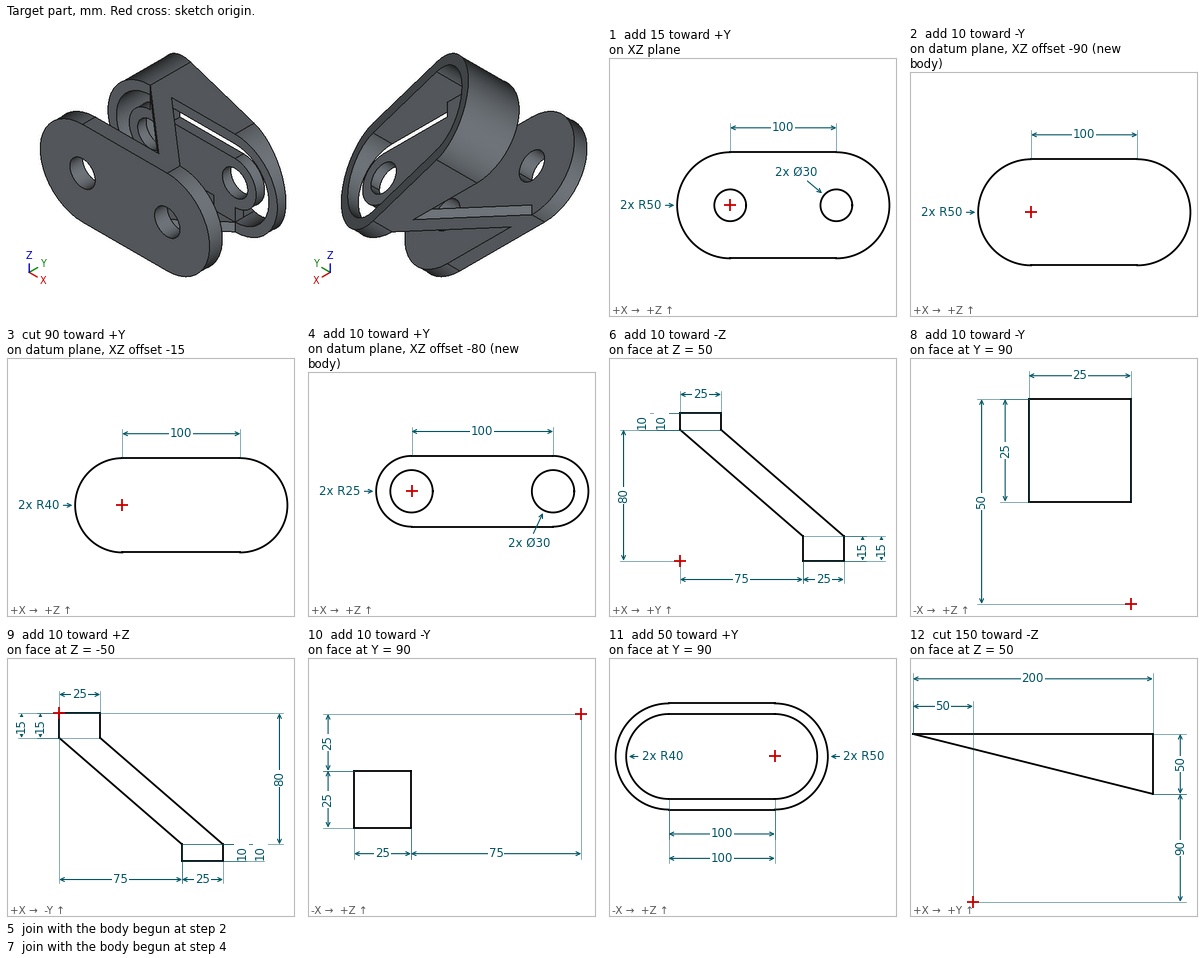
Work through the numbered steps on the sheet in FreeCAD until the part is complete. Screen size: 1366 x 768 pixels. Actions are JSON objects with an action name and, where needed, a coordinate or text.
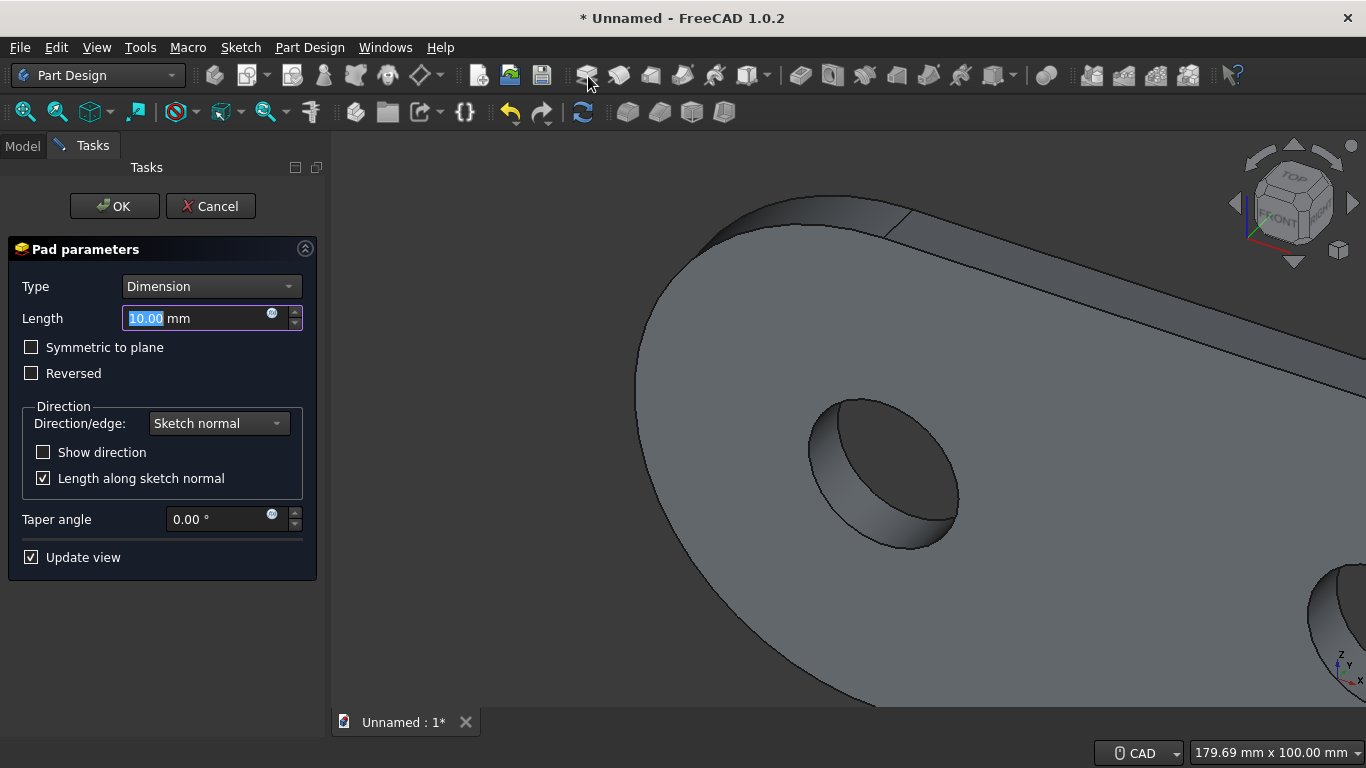
{"action": "type", "text": "15"}
{"action": "key", "text": "Tab"}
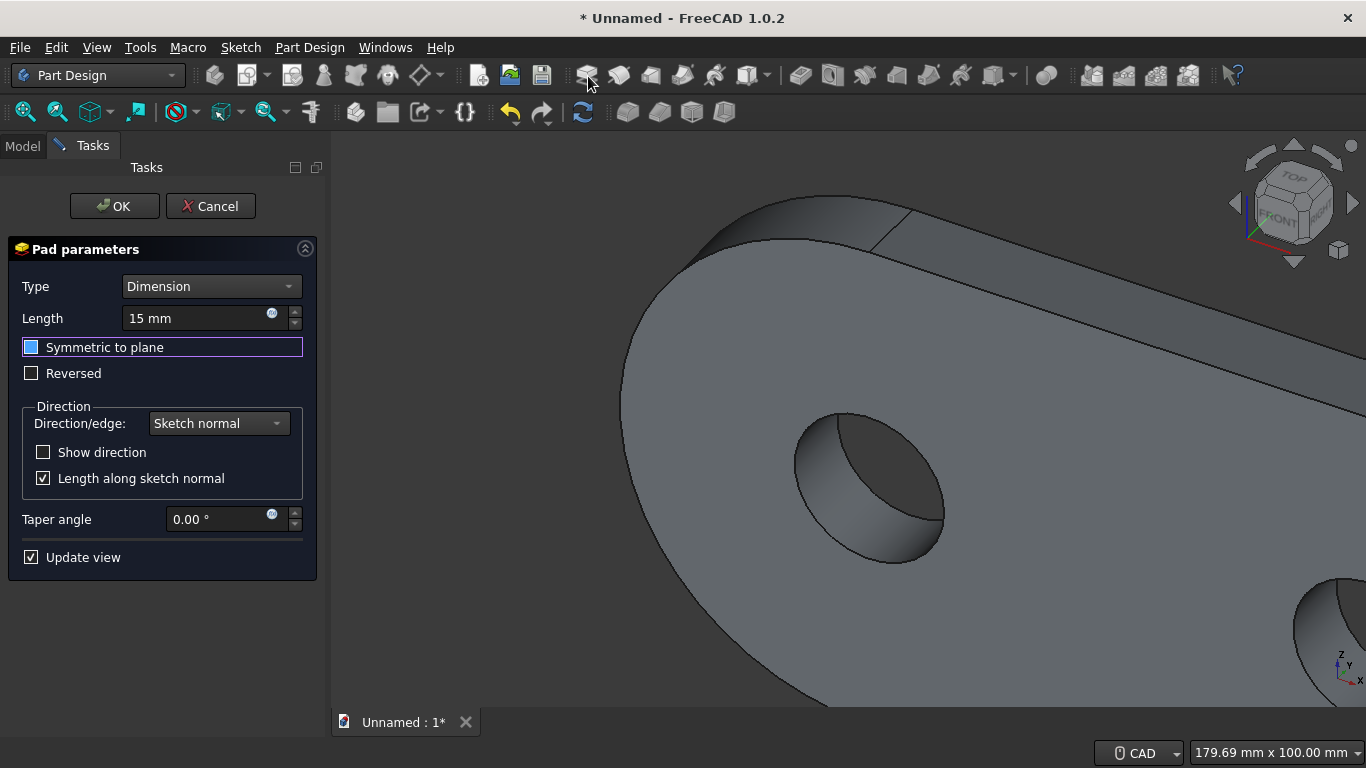
{"action": "left_click", "coordinate": [30, 373]}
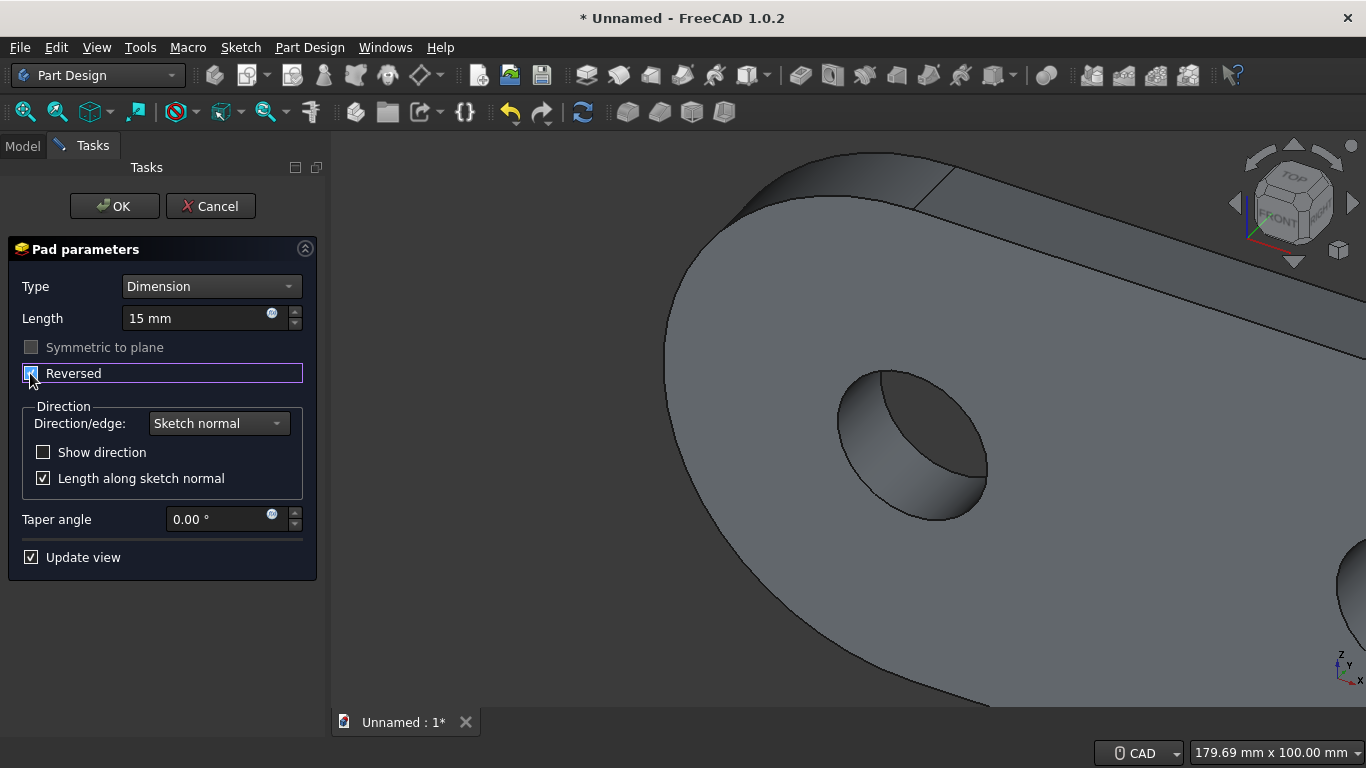
{"action": "left_click", "coordinate": [115, 206]}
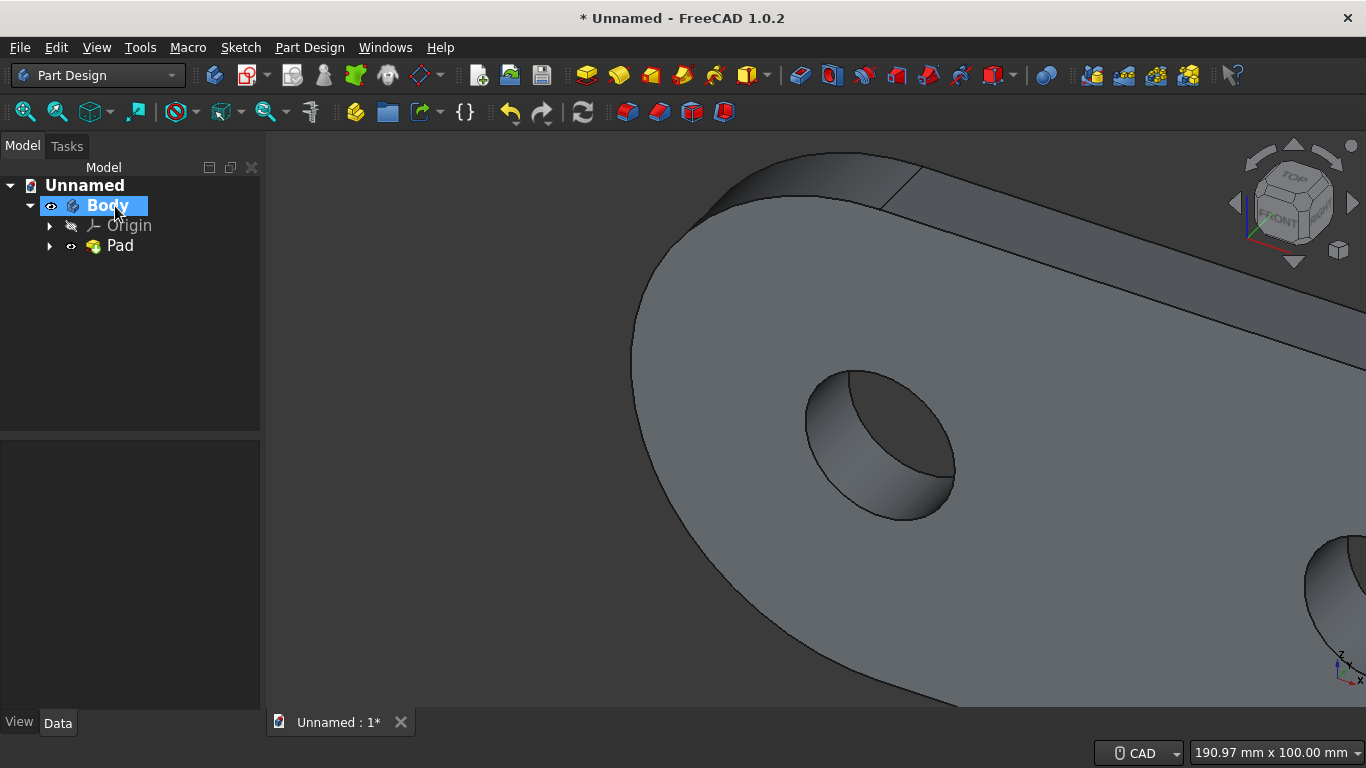
{"action": "left_click", "coordinate": [26, 112]}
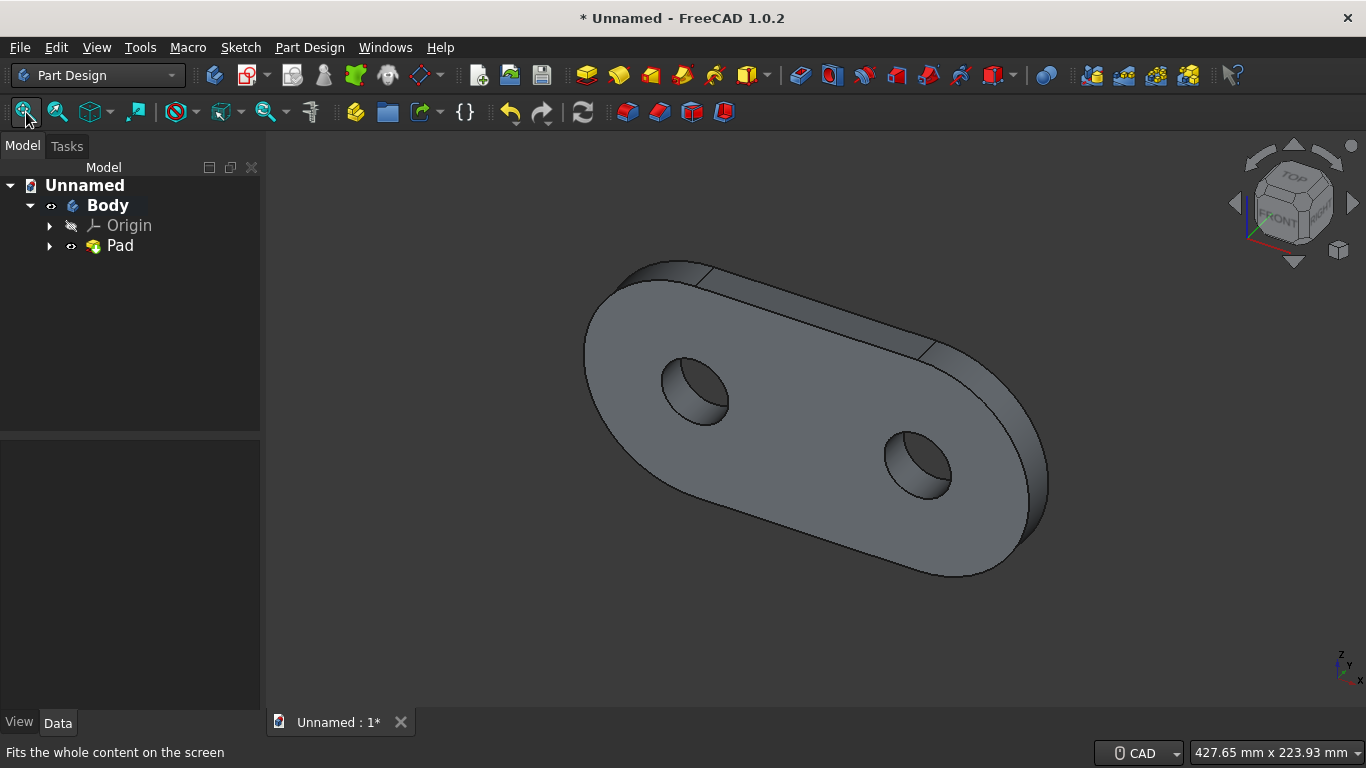
{"action": "left_click", "coordinate": [216, 76]}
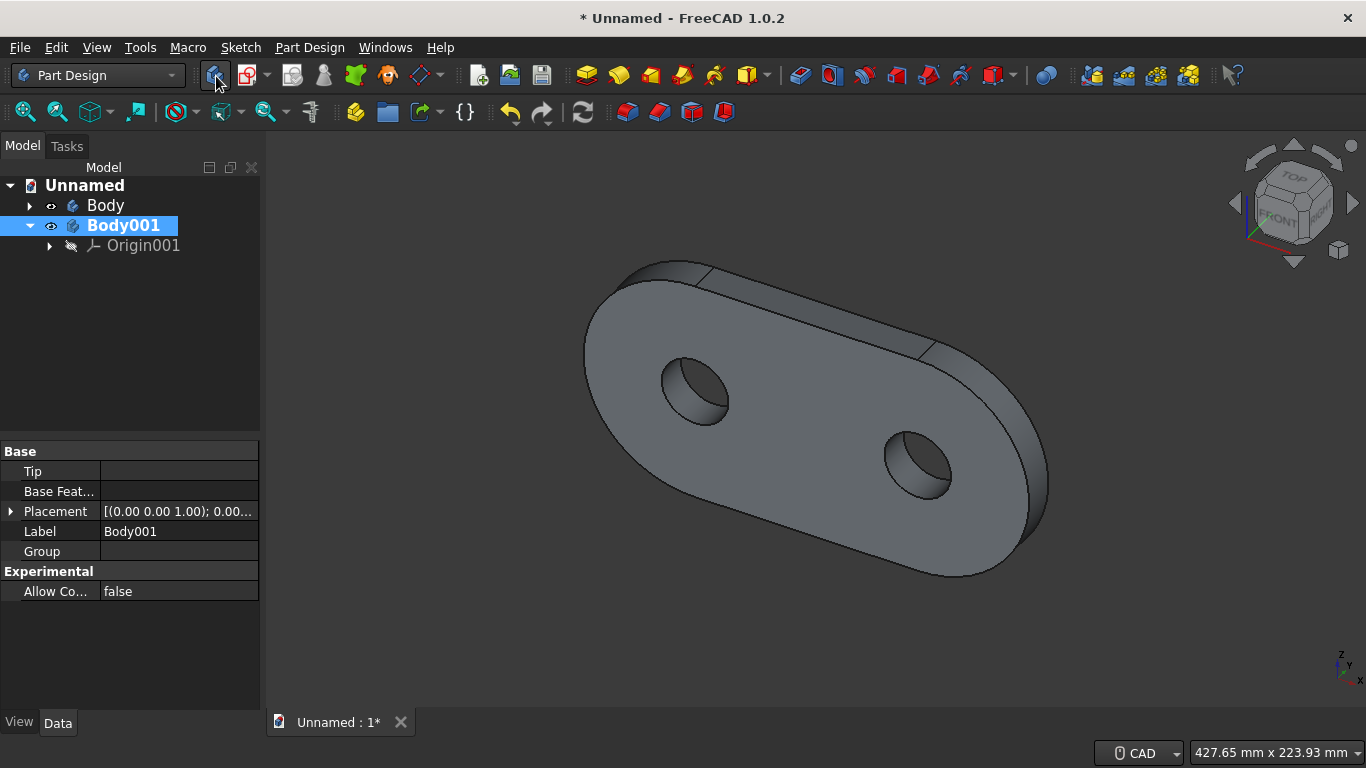
{"action": "left_click", "coordinate": [50, 246]}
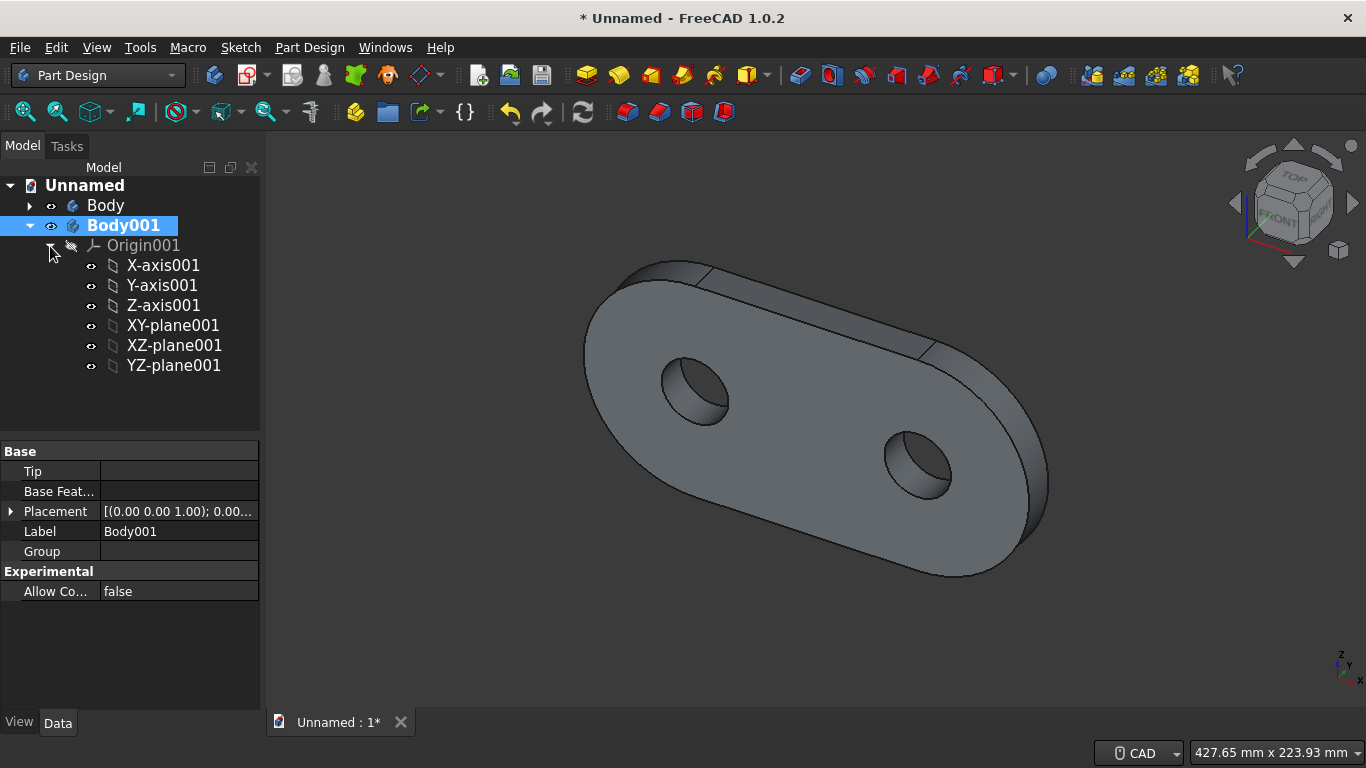
{"action": "left_click", "coordinate": [136, 346]}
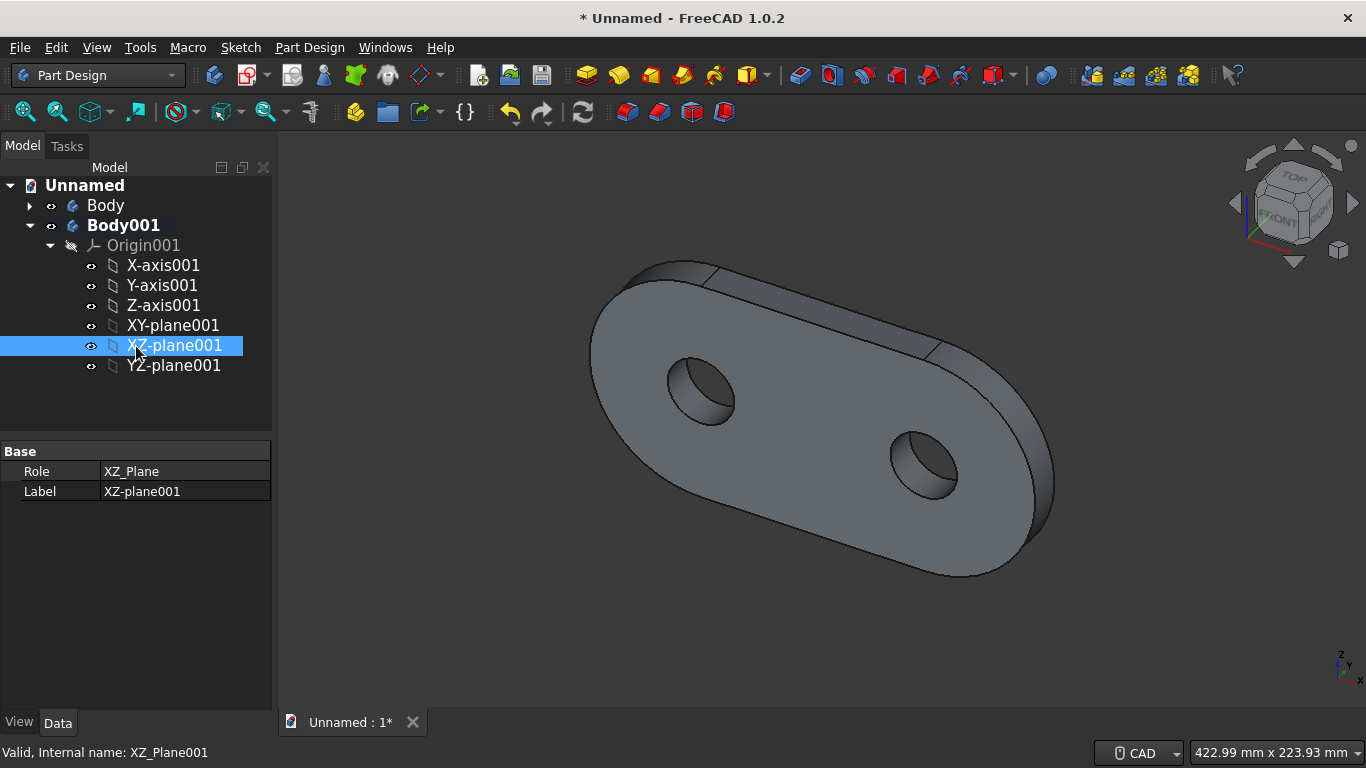
{"action": "left_click", "coordinate": [420, 76]}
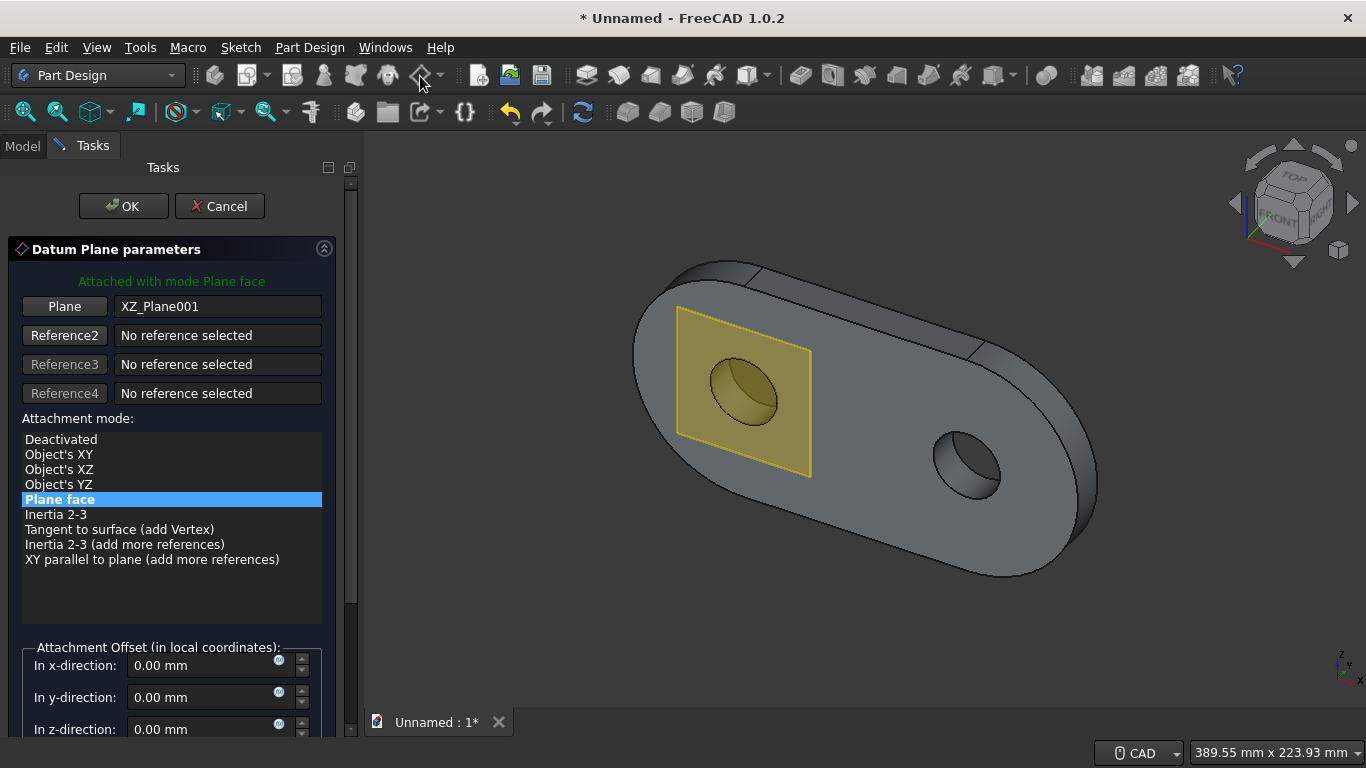
{"action": "scroll", "coordinate": [351, 456], "scroll_direction": "down", "scroll_amount": 2}